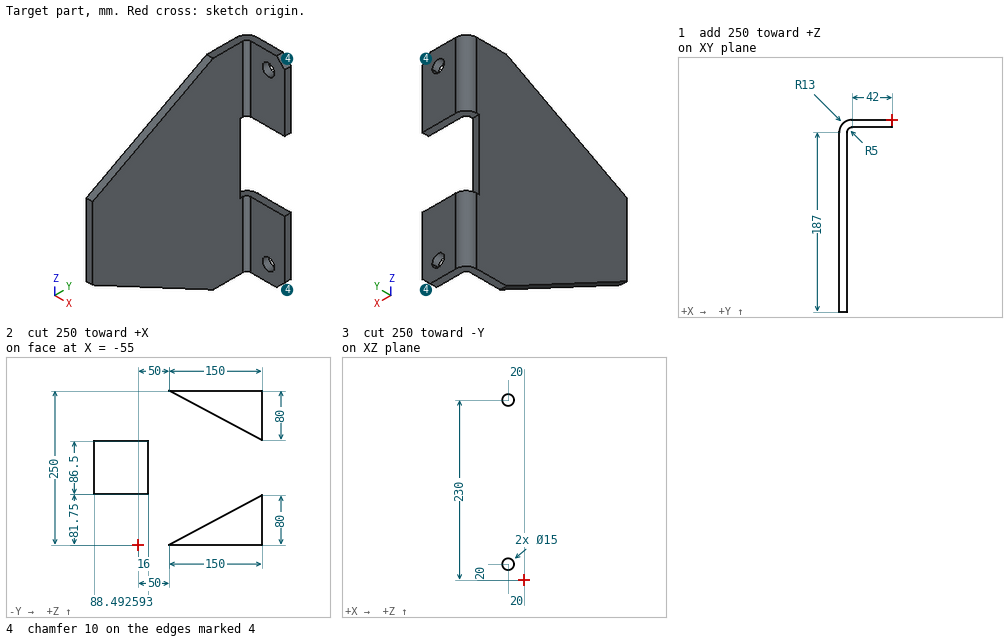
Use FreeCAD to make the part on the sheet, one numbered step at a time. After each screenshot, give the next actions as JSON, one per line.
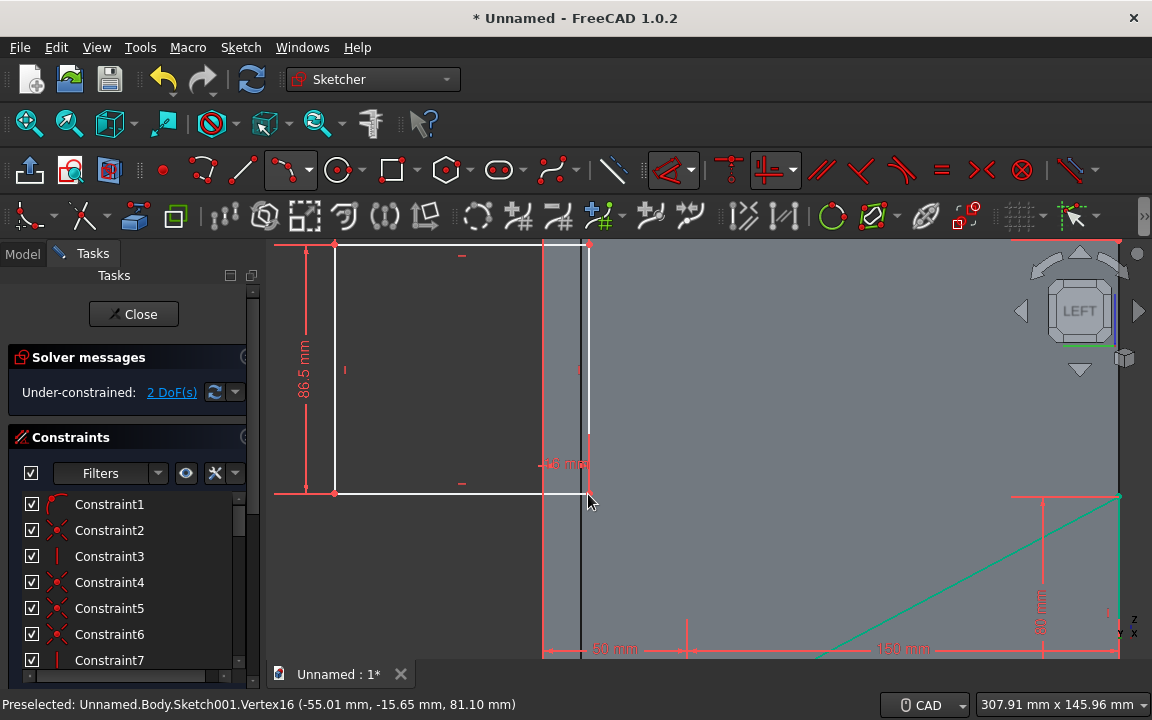
{"action": "scroll", "coordinate": [590, 496], "scroll_direction": "down", "scroll_amount": 5}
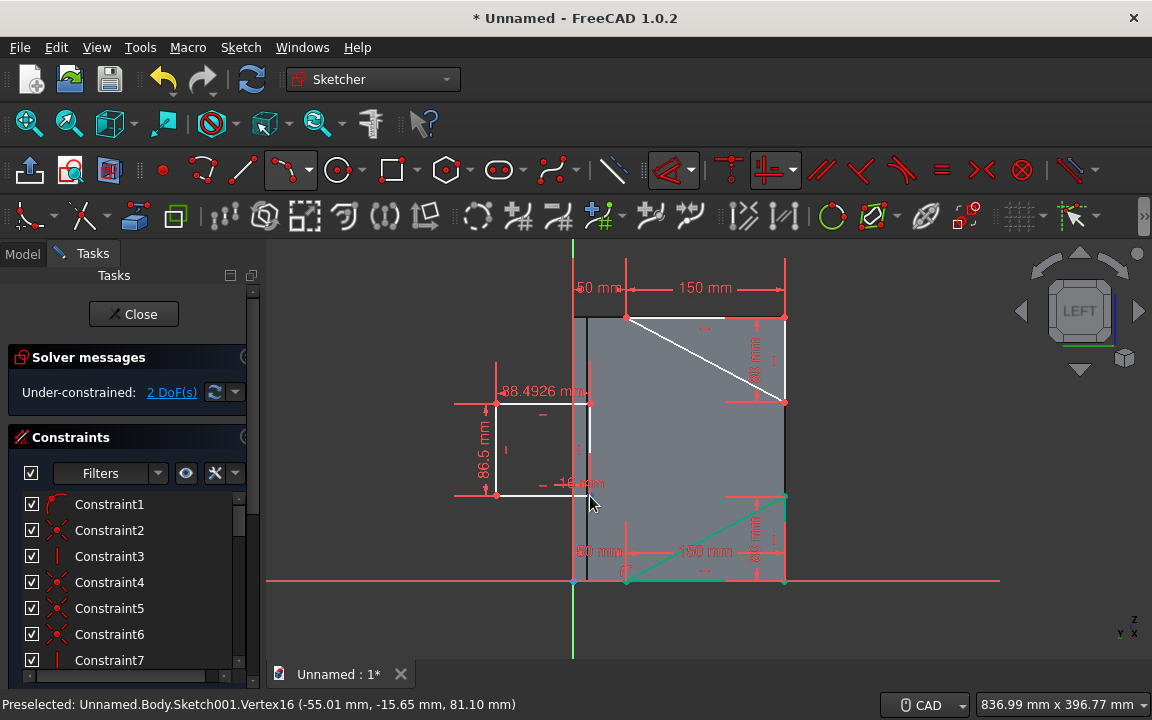
{"action": "left_click", "coordinate": [626, 318]}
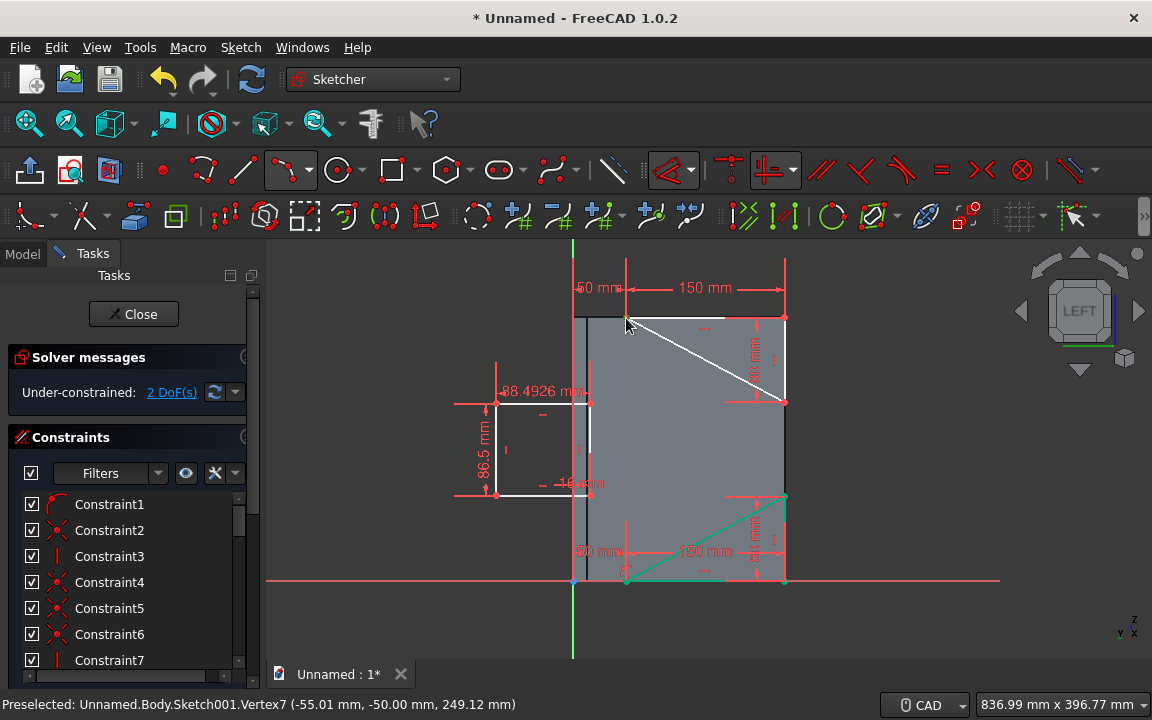
{"action": "left_click", "coordinate": [694, 170]}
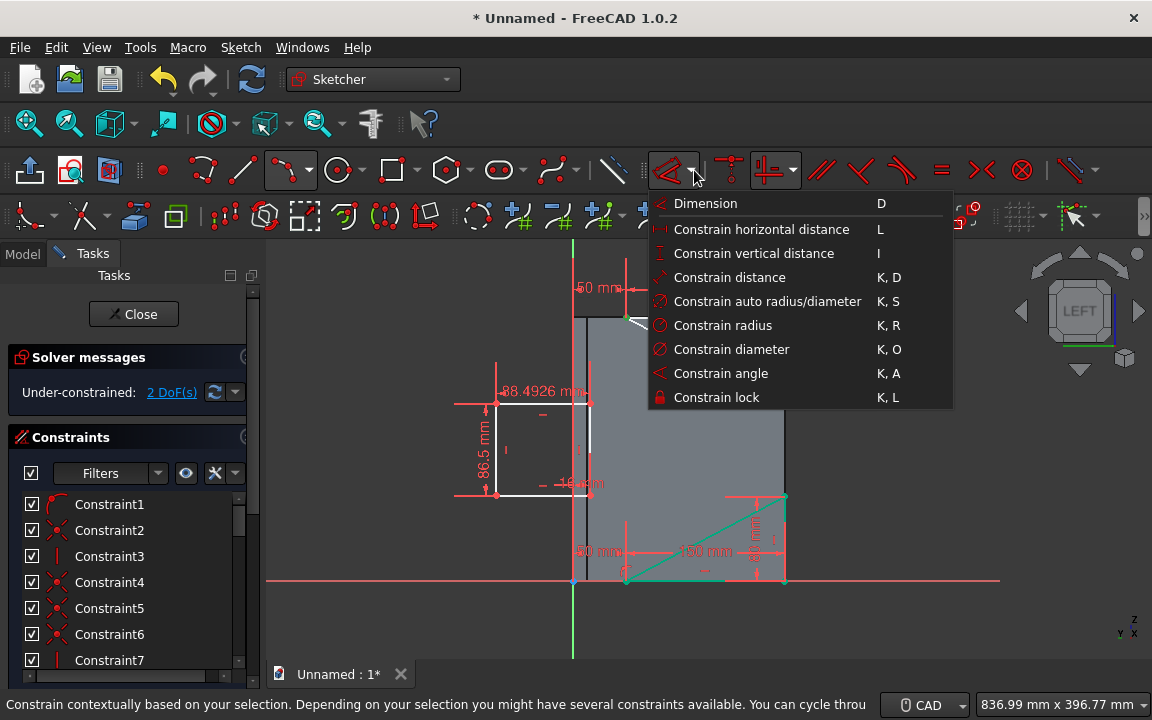
{"action": "left_click", "coordinate": [801, 253]}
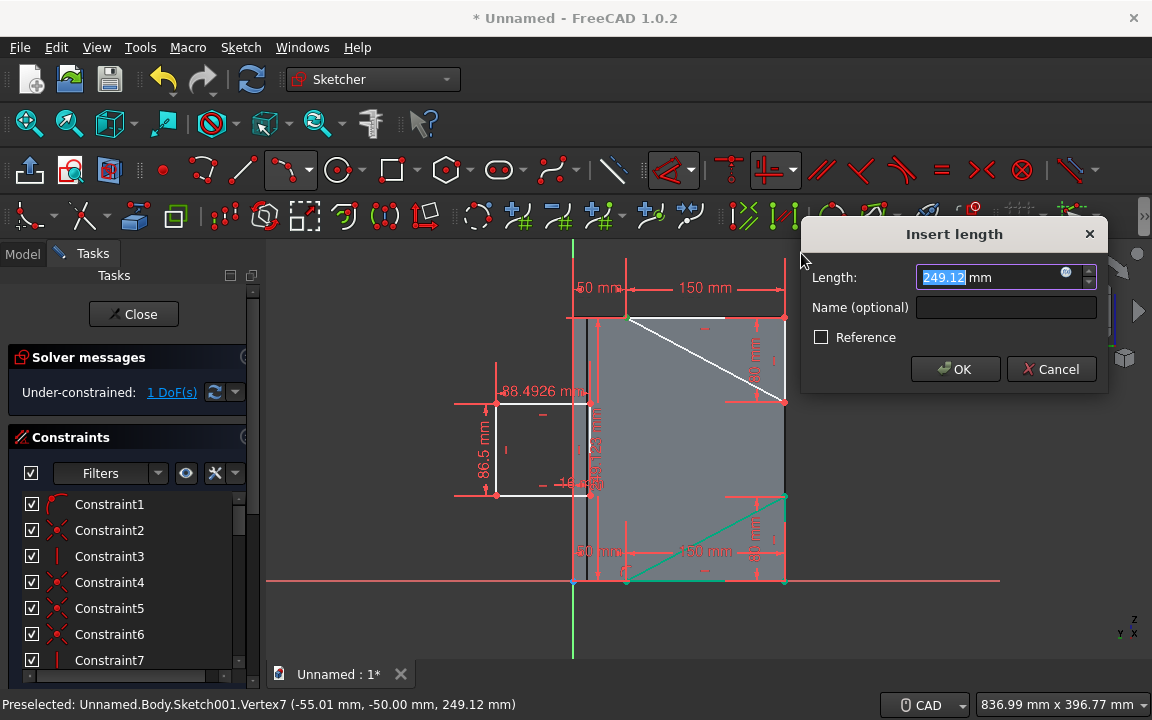
{"action": "type", "text": "250"}
{"action": "key", "text": "Return"}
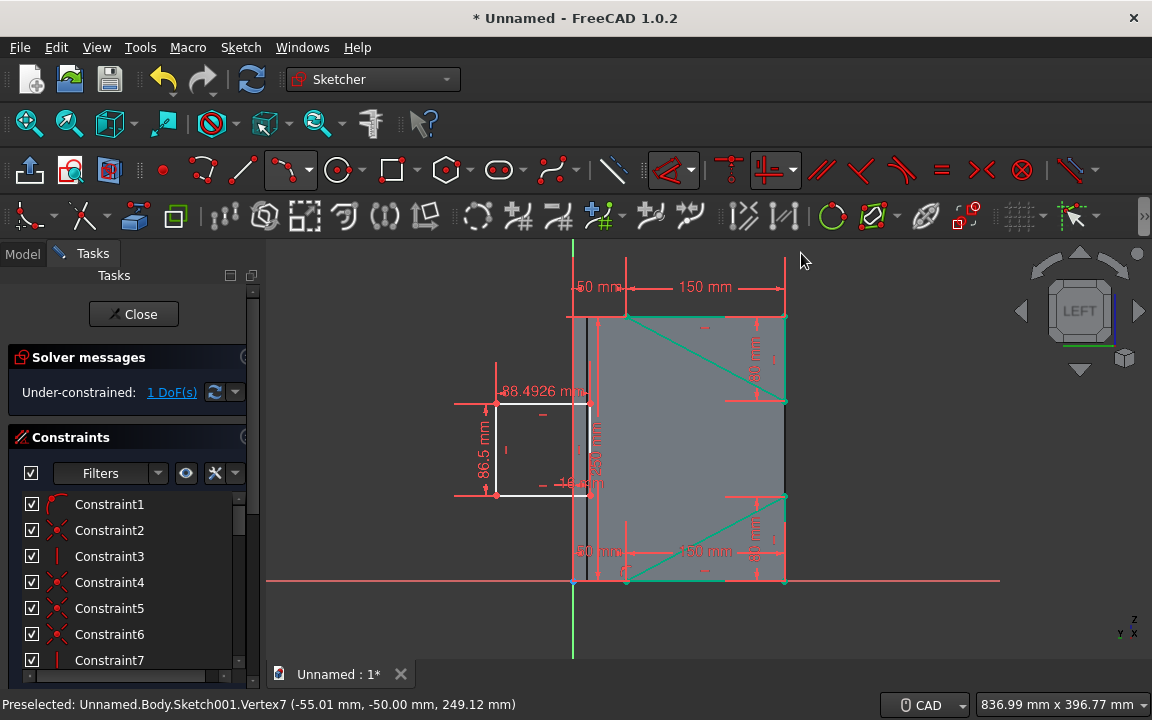
{"action": "left_click", "coordinate": [496, 496]}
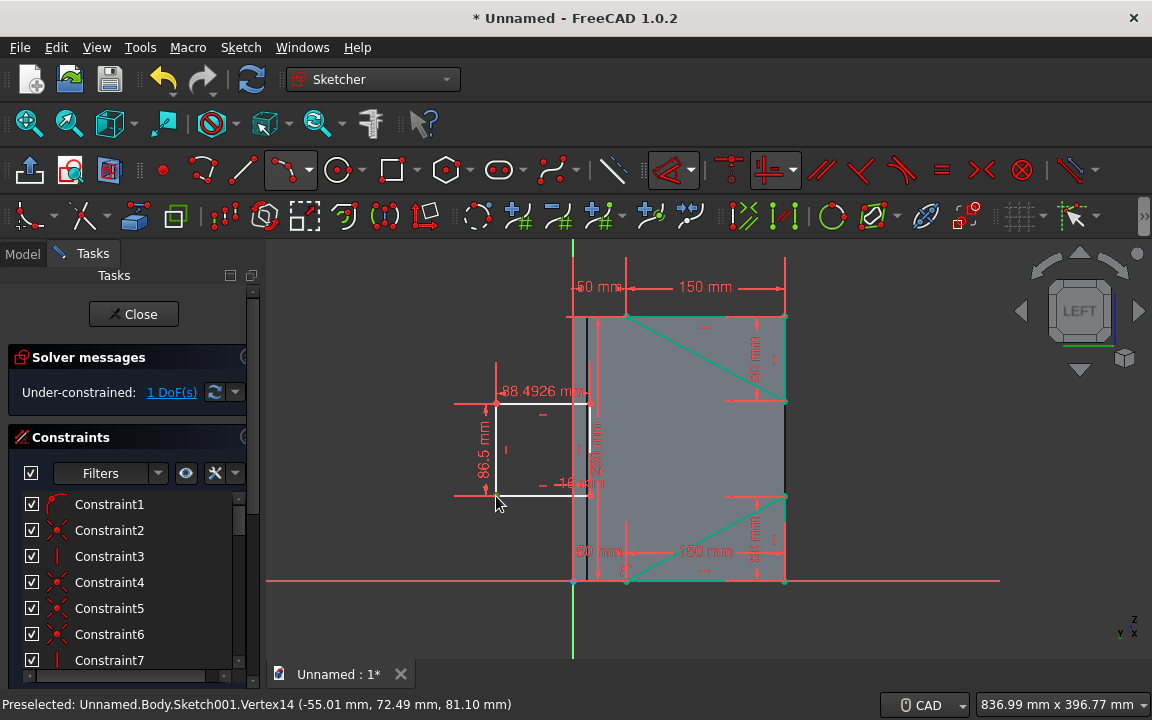
{"action": "key", "text": "i"}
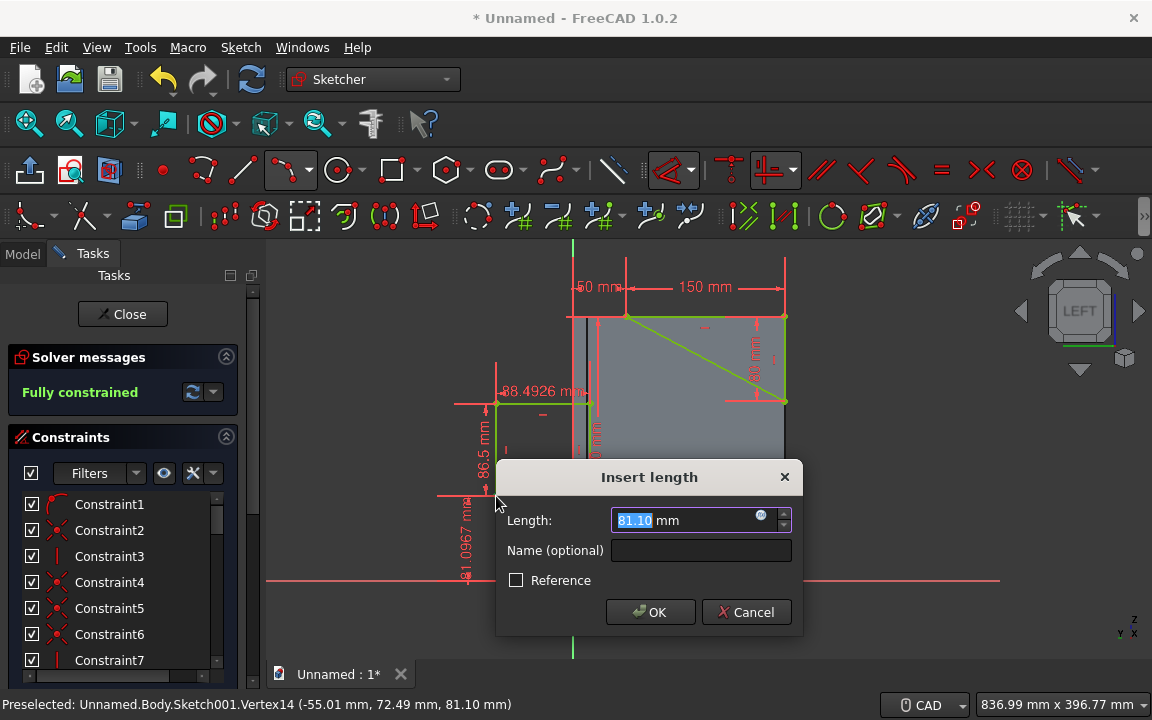
{"action": "type", "text": "81.75"}
{"action": "key", "text": "Return"}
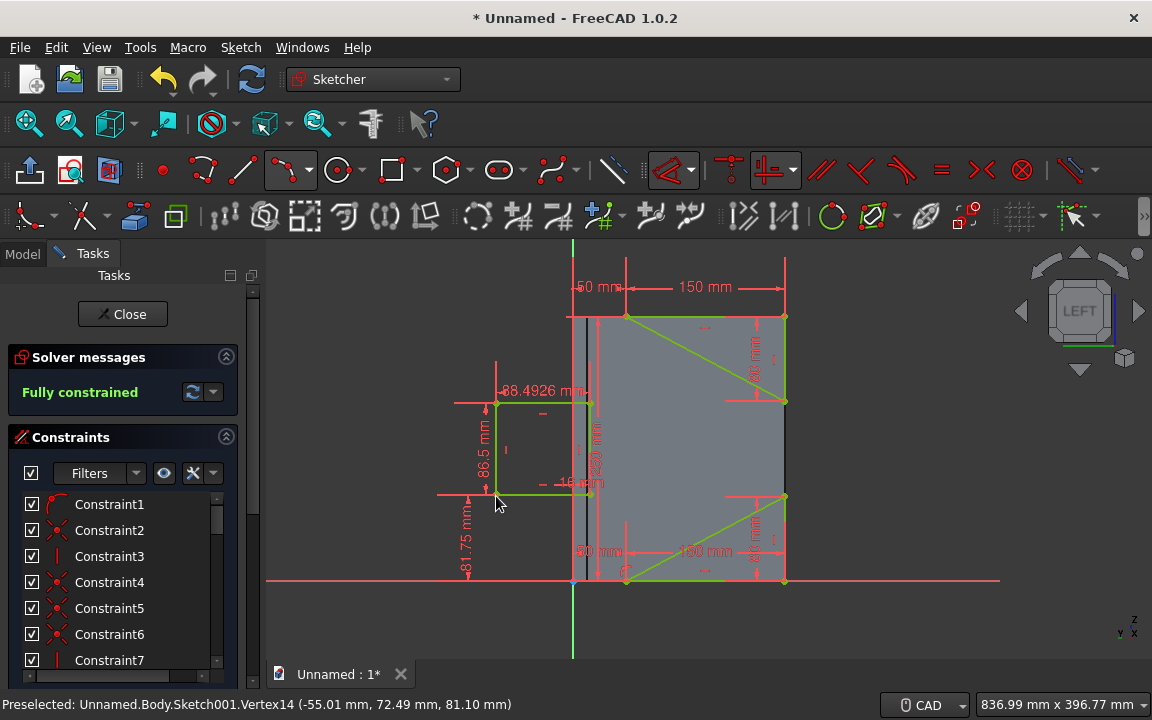
{"action": "left_click", "coordinate": [123, 314]}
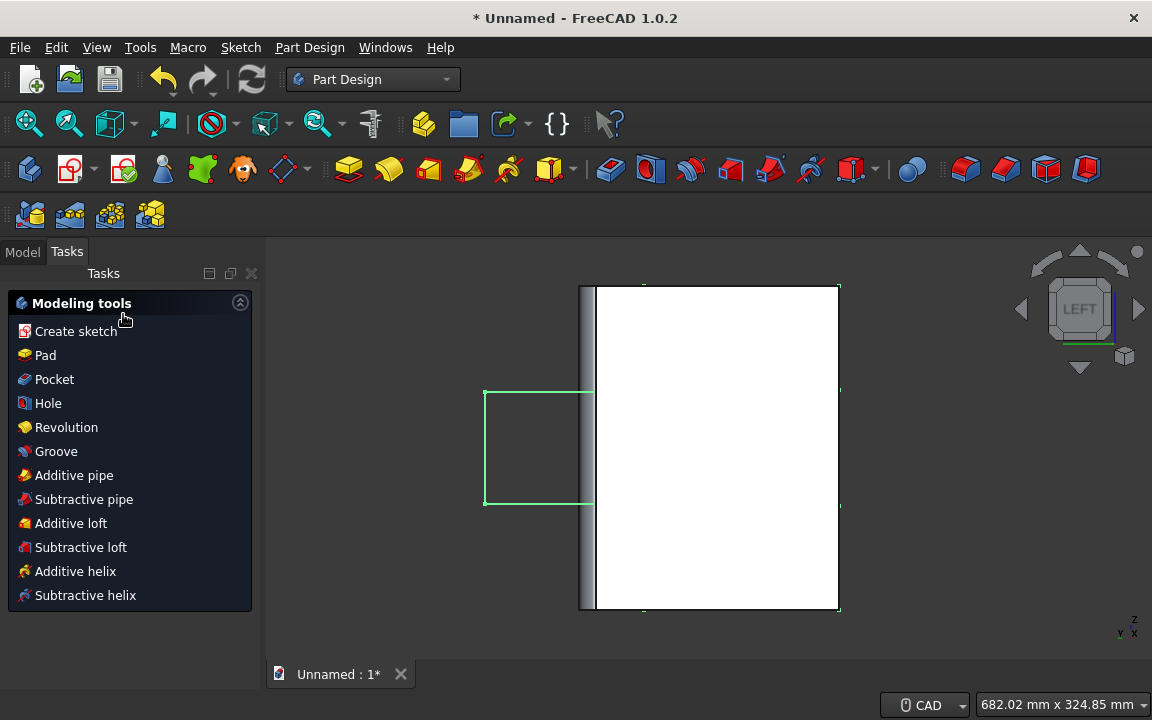
{"action": "left_click", "coordinate": [612, 170]}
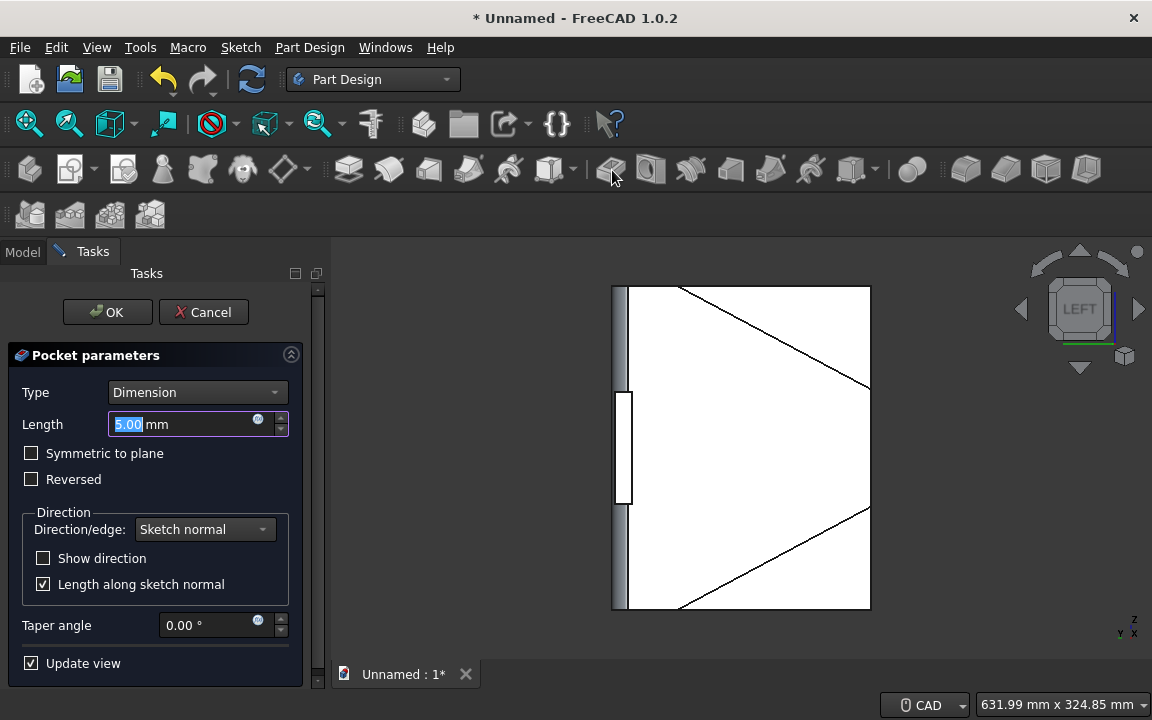
{"action": "type", "text": "250"}
{"action": "key", "text": "Tab"}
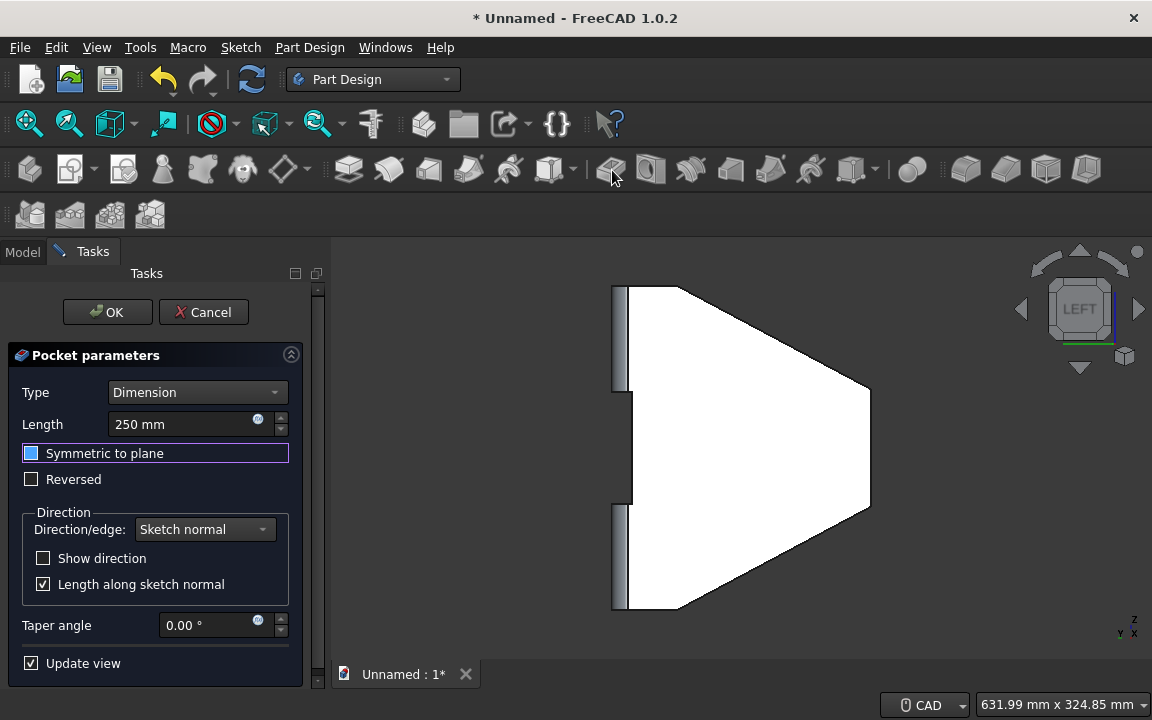
{"action": "left_click", "coordinate": [108, 312]}